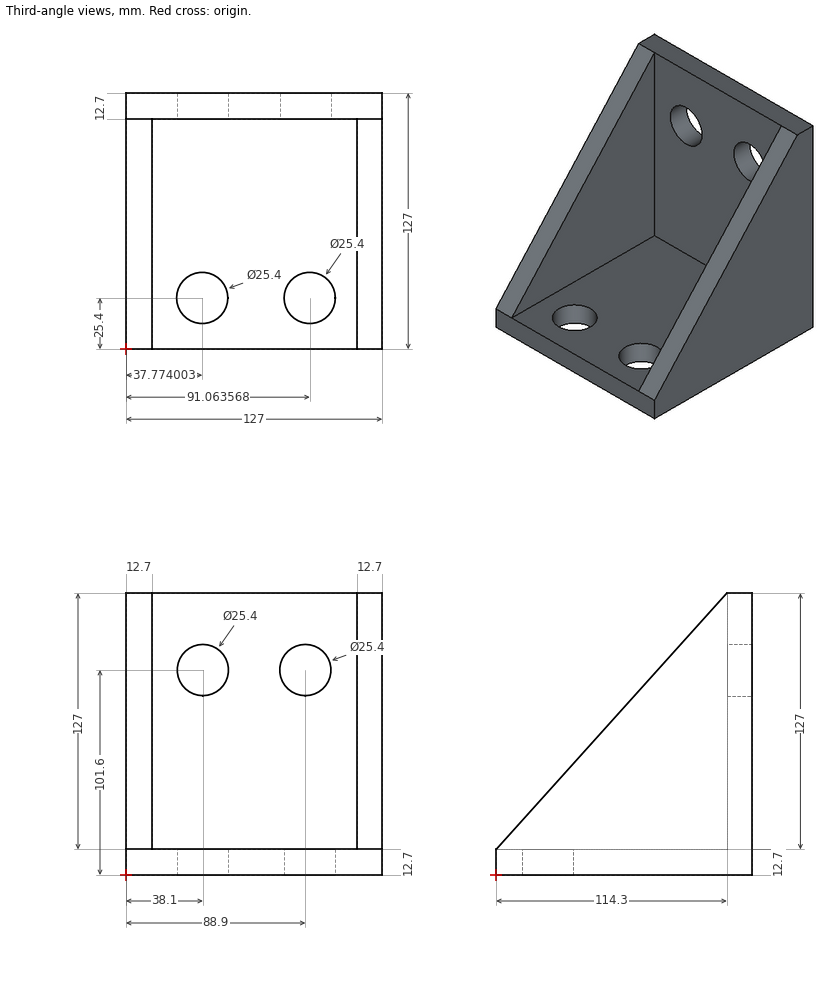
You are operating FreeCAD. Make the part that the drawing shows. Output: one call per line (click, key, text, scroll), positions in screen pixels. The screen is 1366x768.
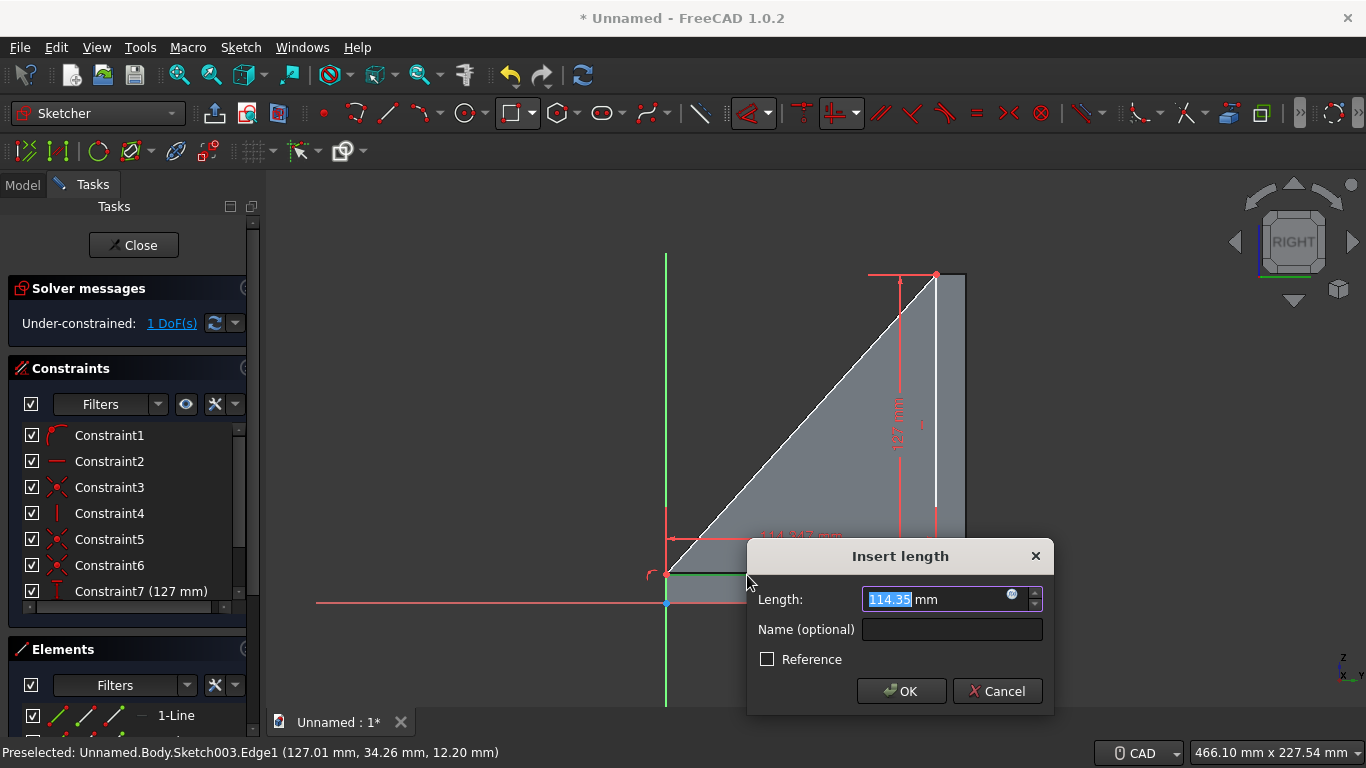
text(114.3)
key(Return)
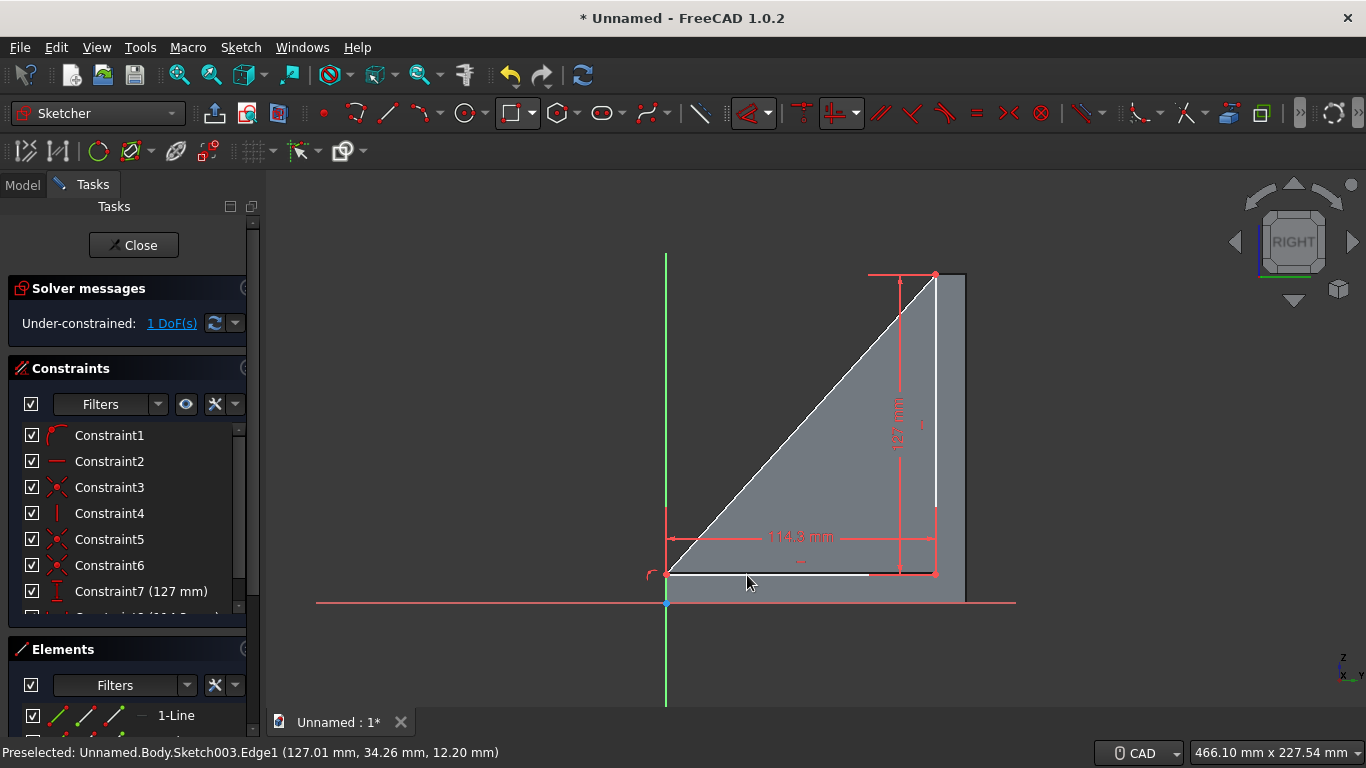
scroll(666, 575, up, 2)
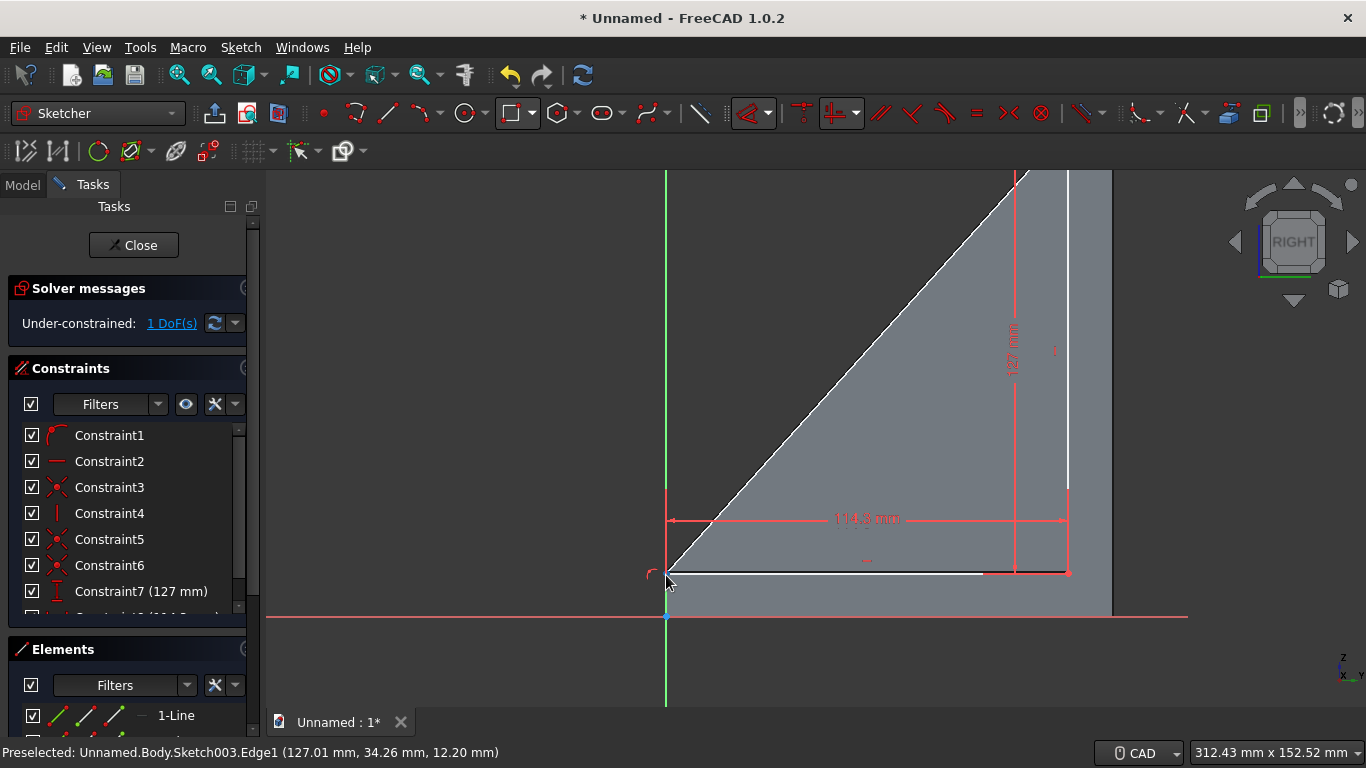
click(666, 574)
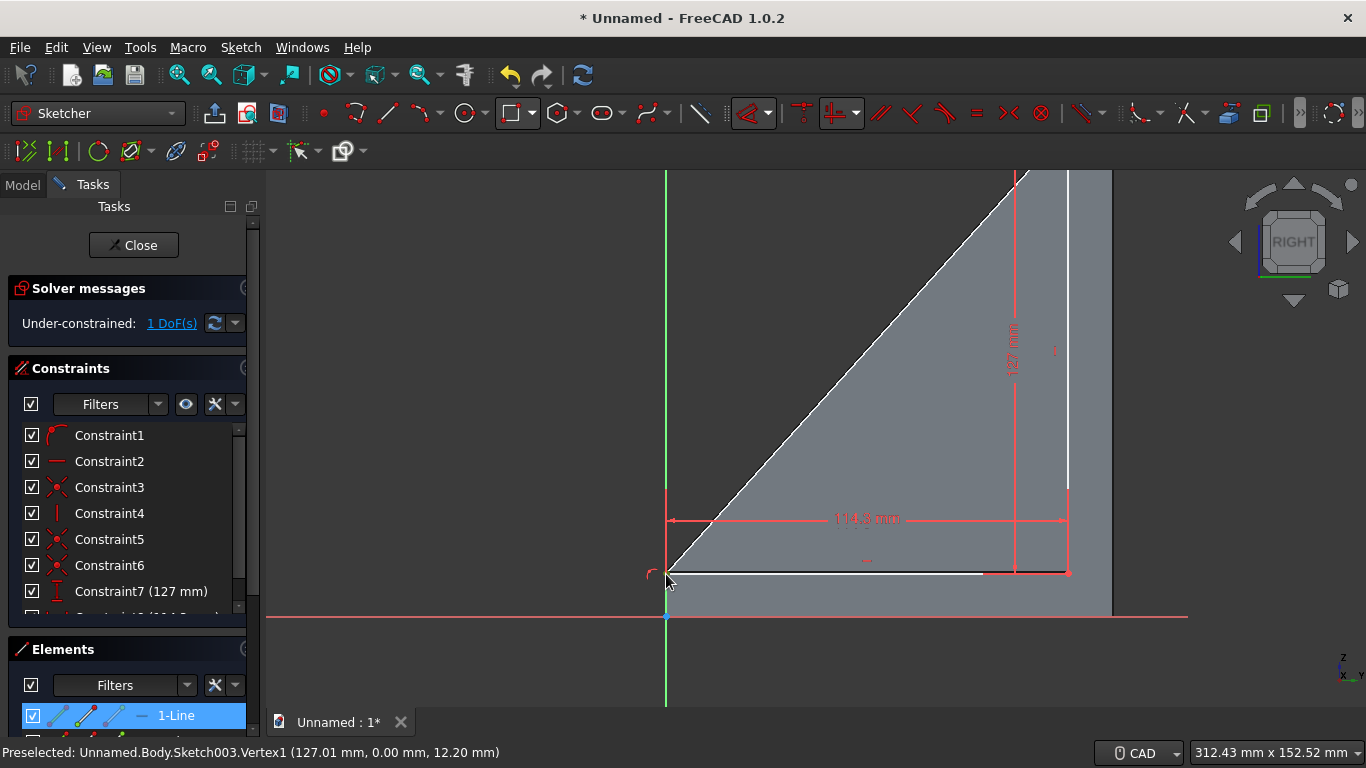
key(i)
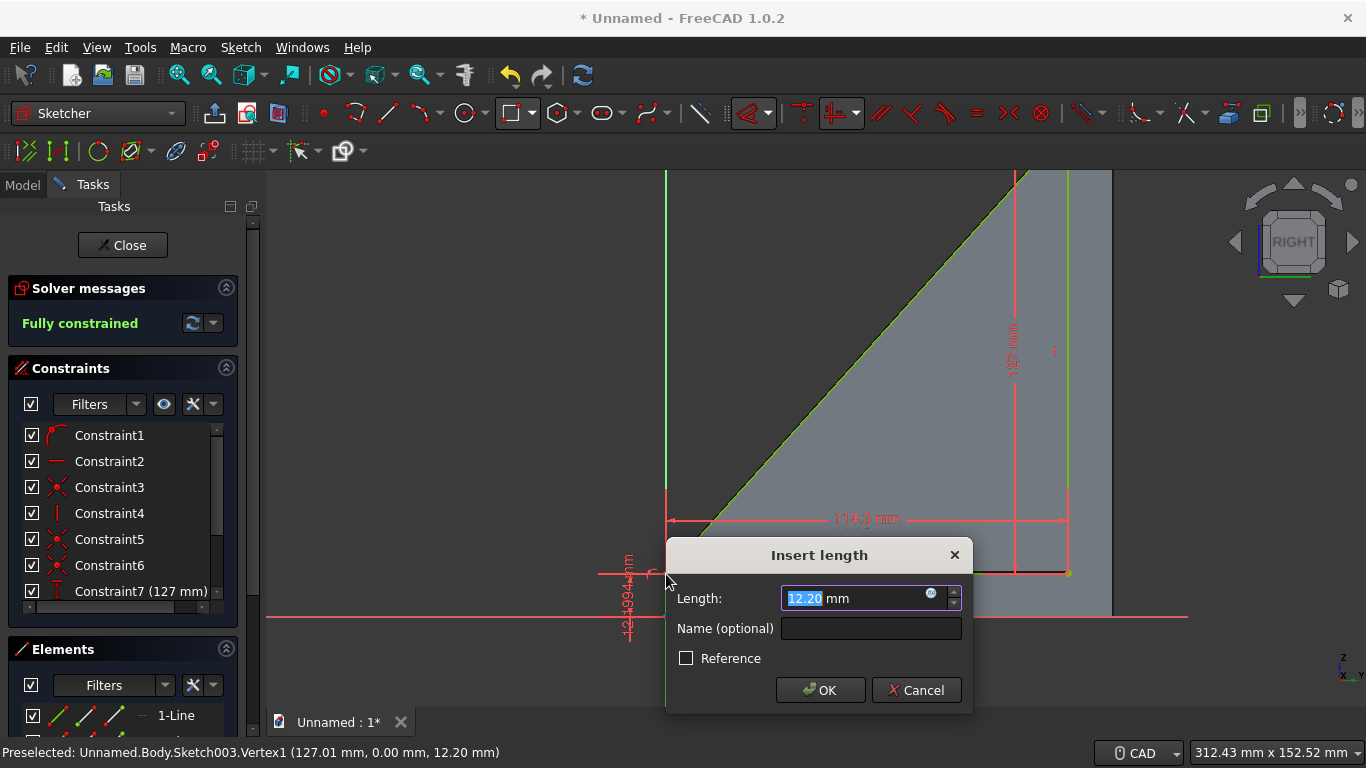
text(12.7)
key(Return)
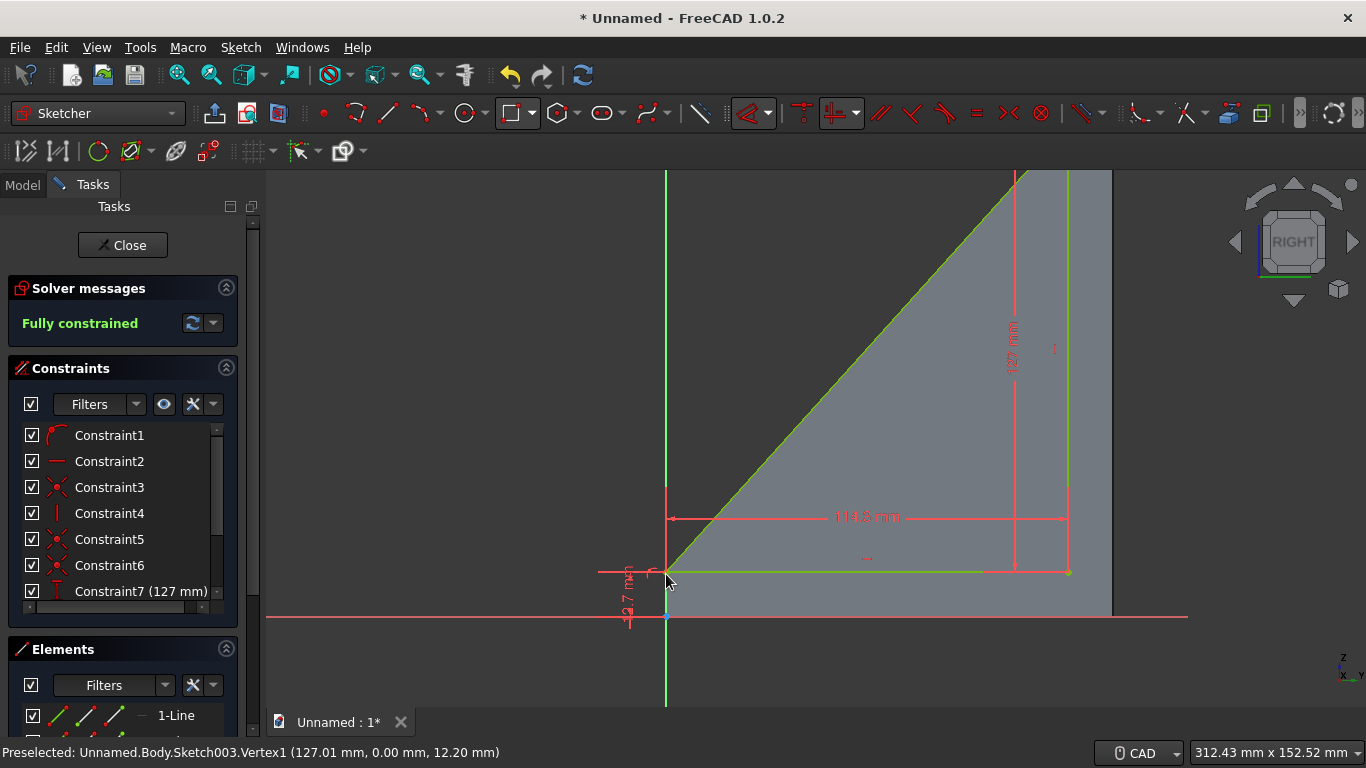
click(123, 245)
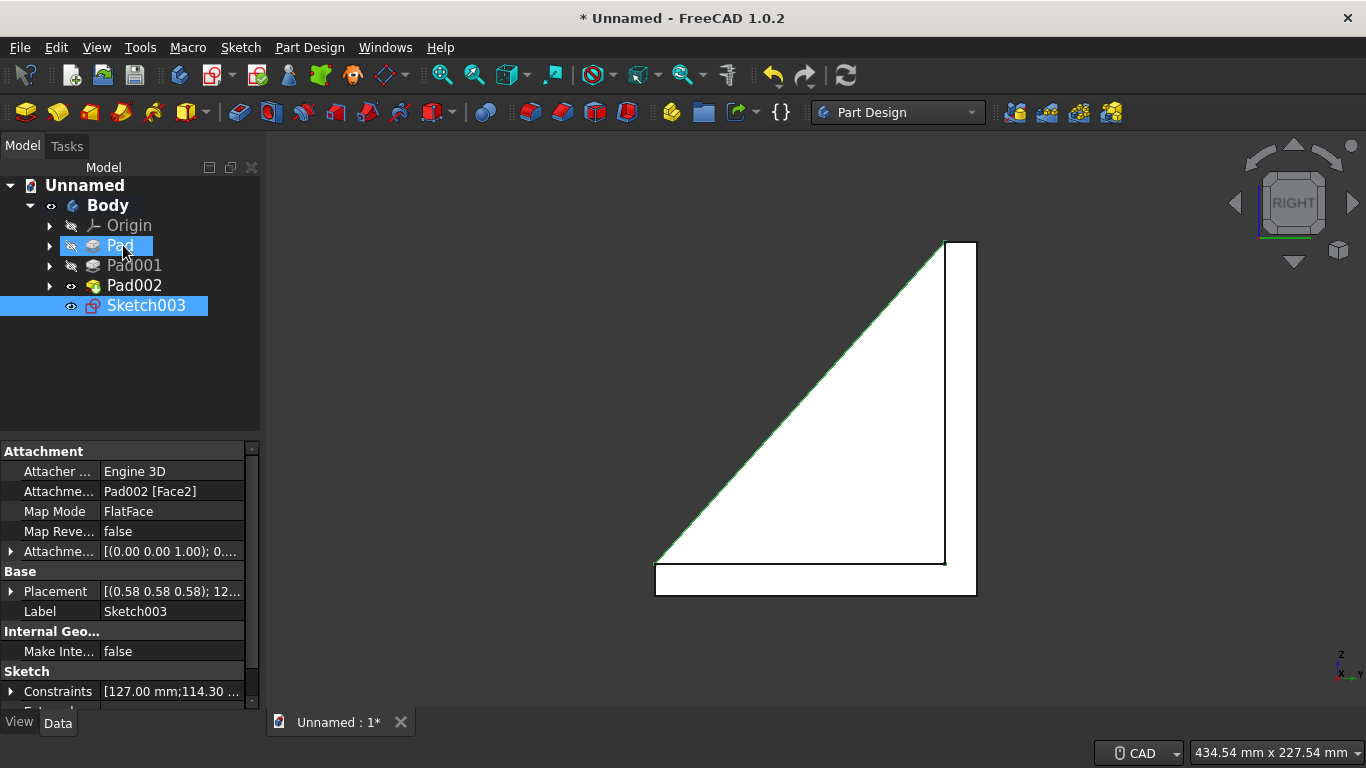
click(26, 112)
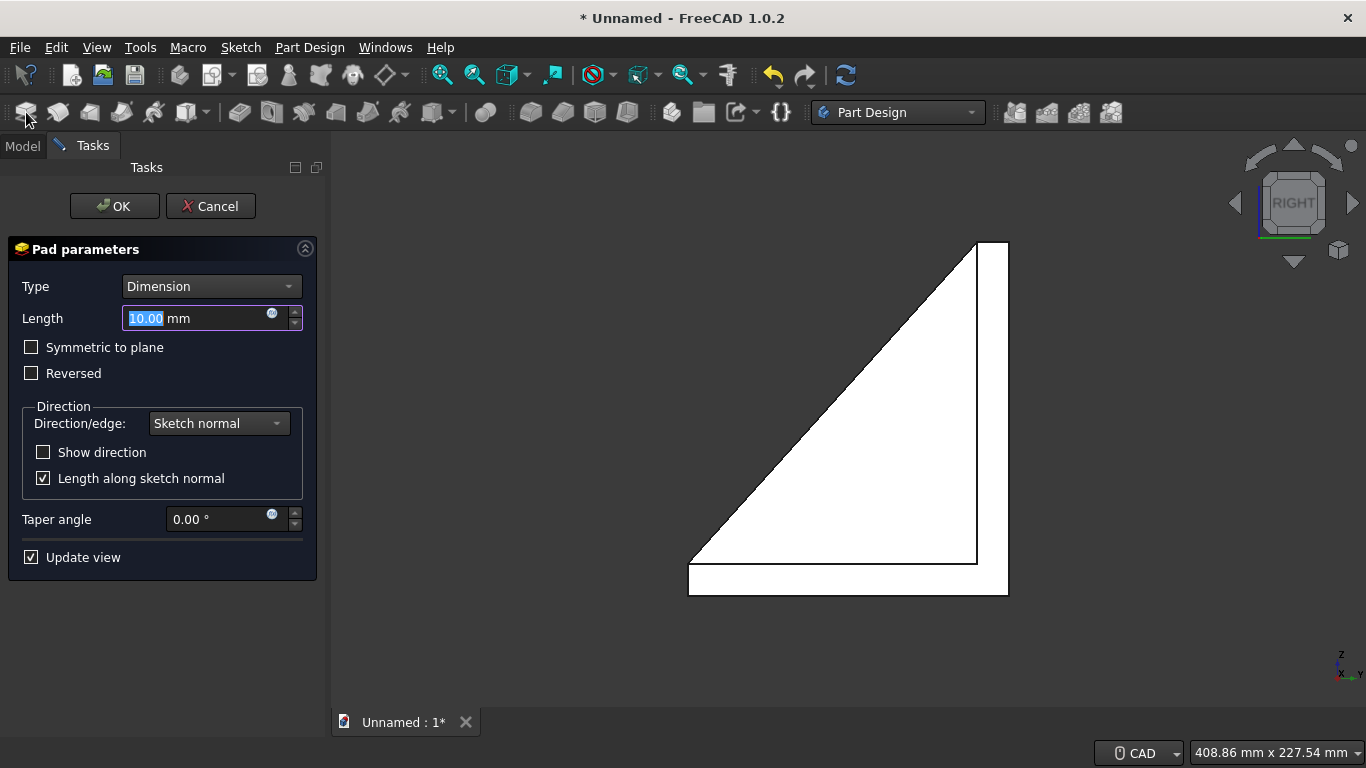
text(12.7)
key(Tab)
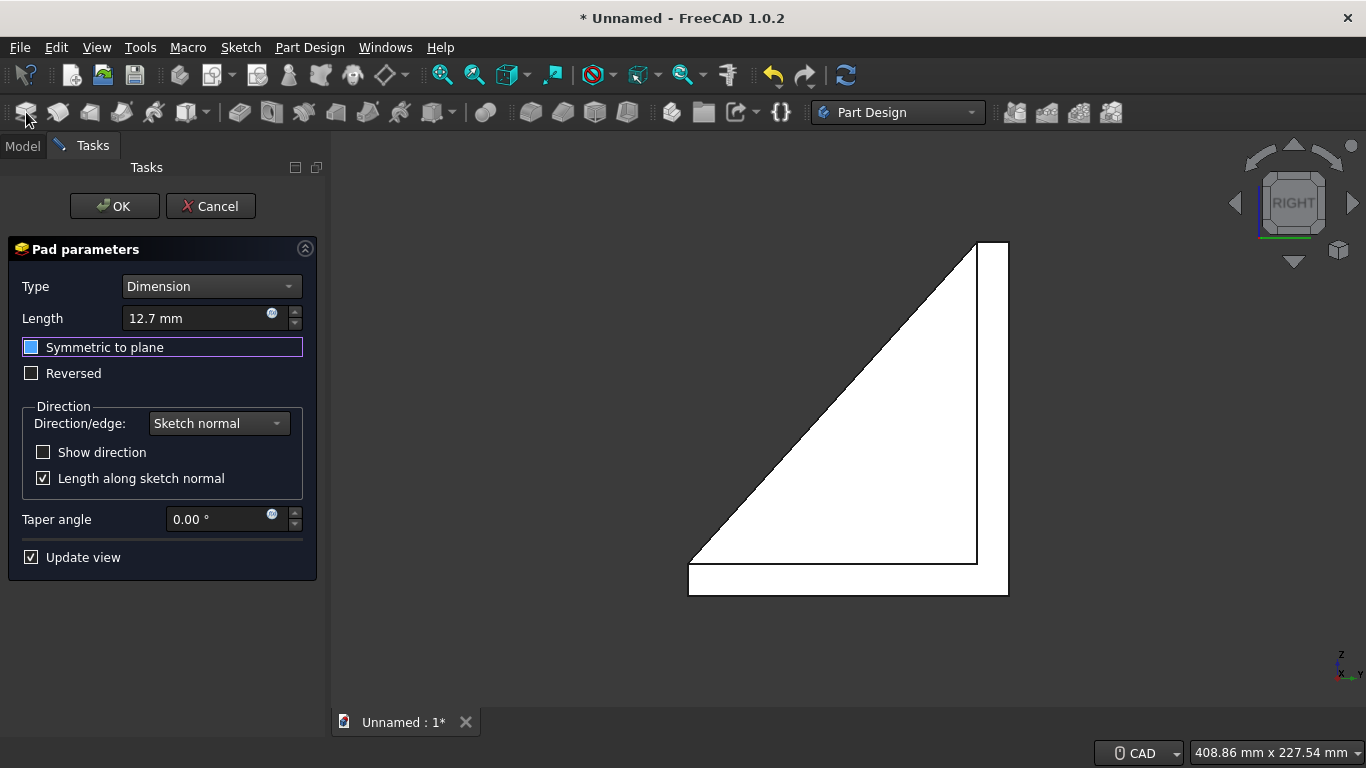
click(30, 373)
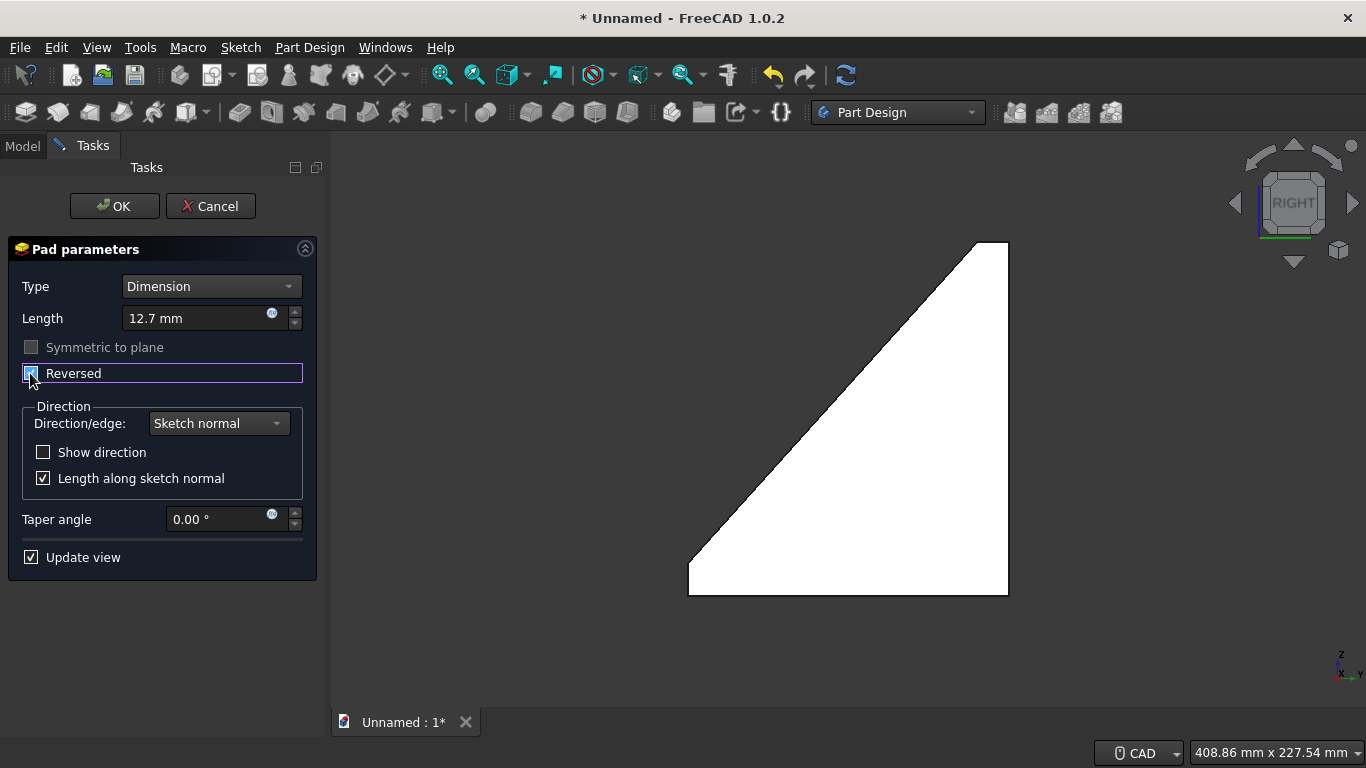
click(115, 206)